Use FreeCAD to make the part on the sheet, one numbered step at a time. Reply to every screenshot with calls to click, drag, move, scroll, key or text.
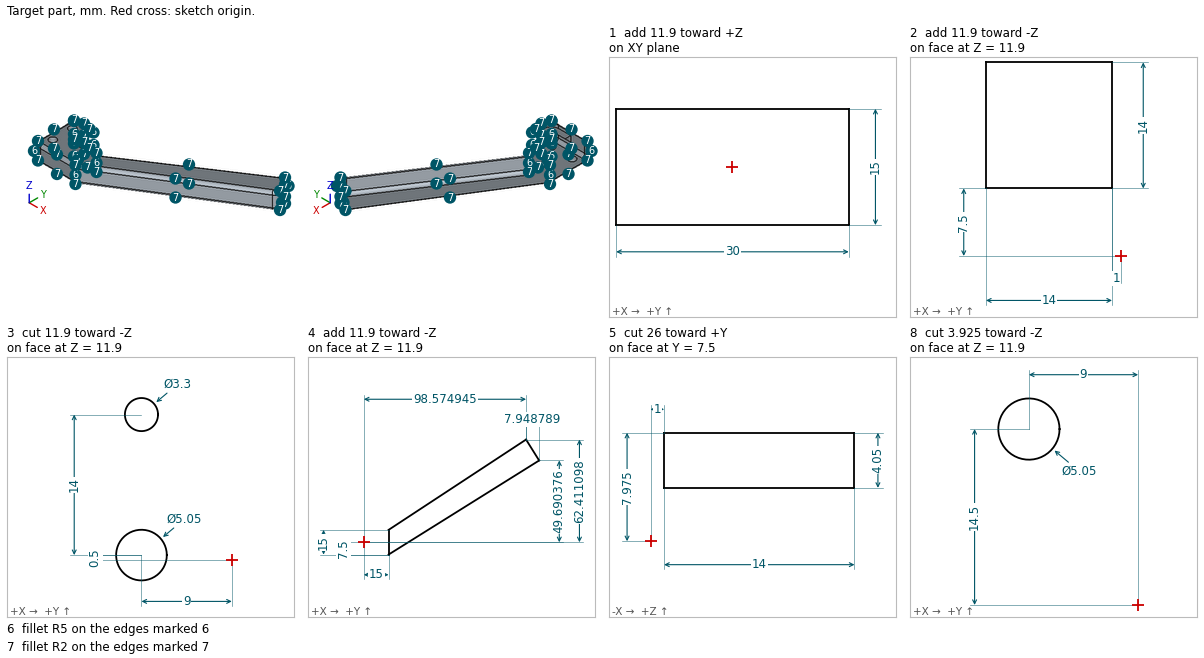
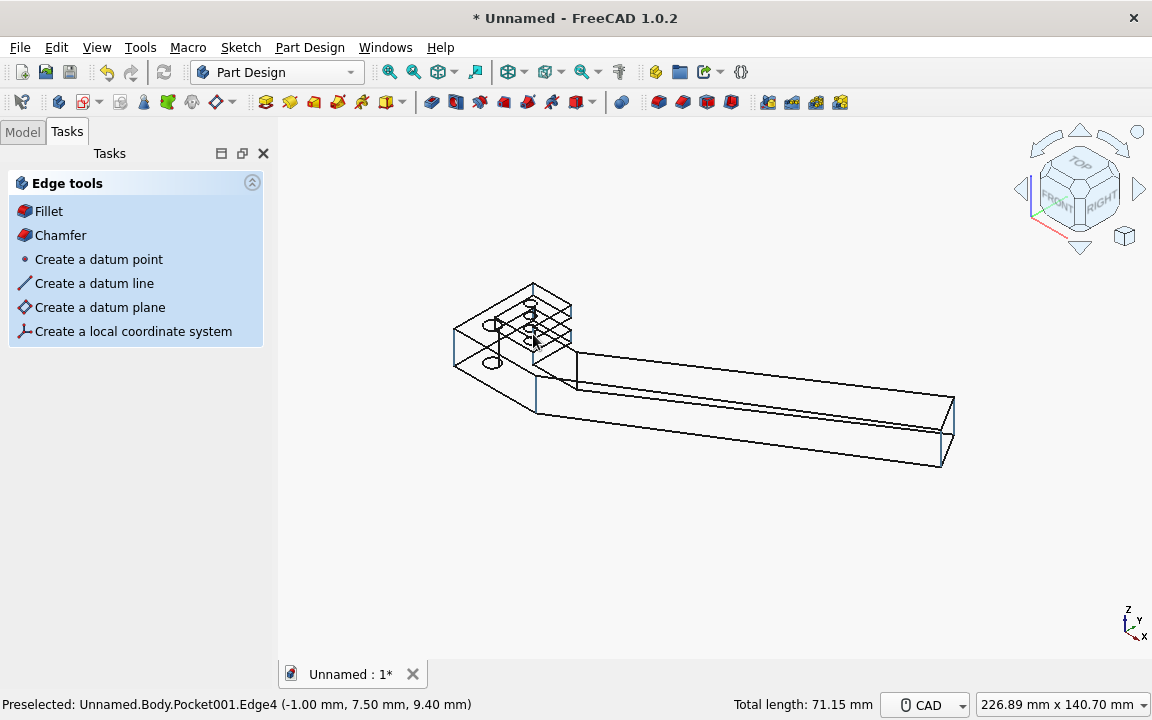
click(577, 370, ctrl)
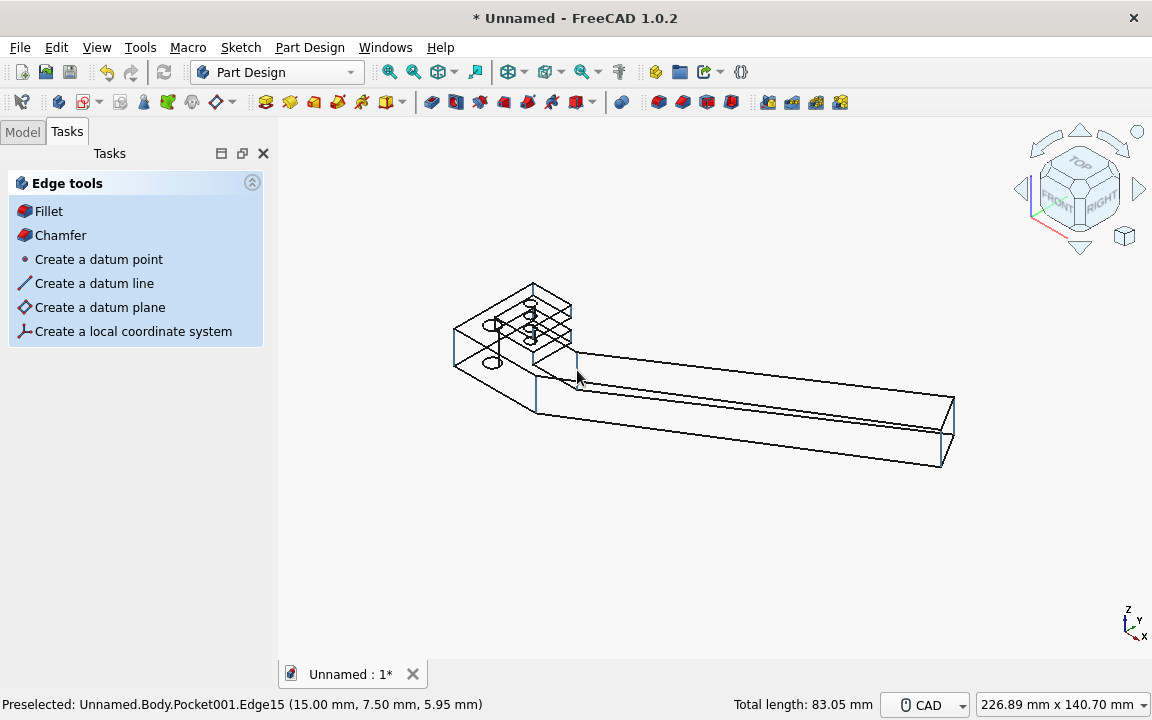
key(v)
key(1)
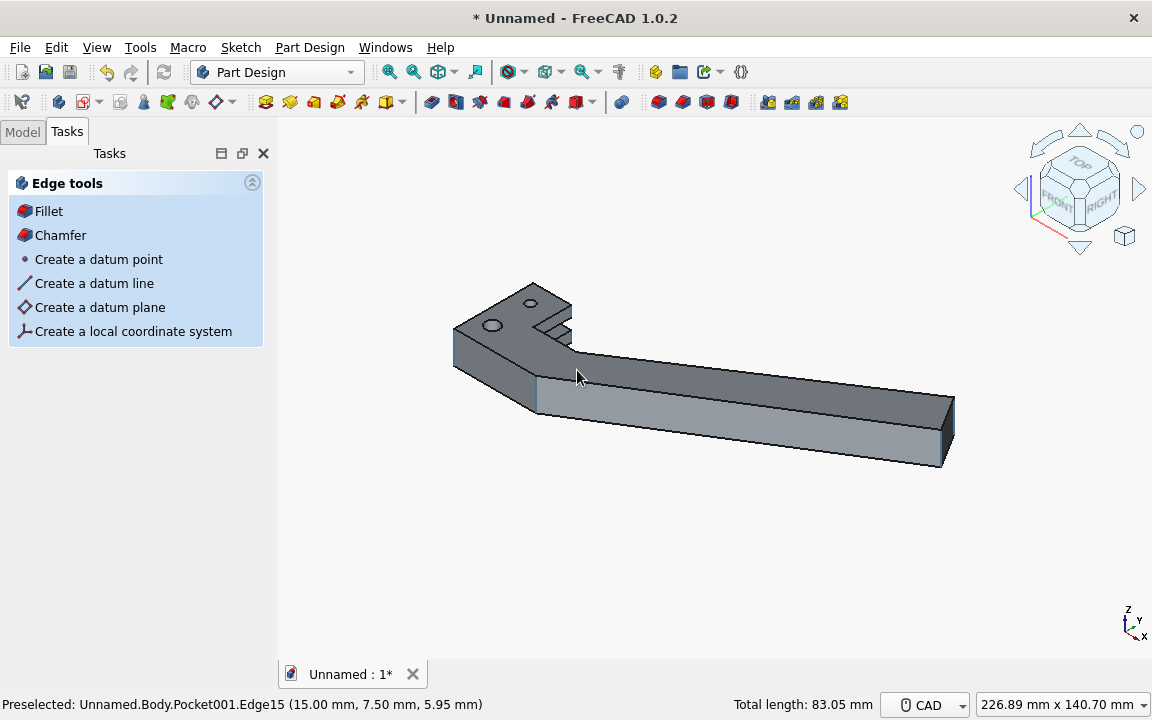
click(660, 102)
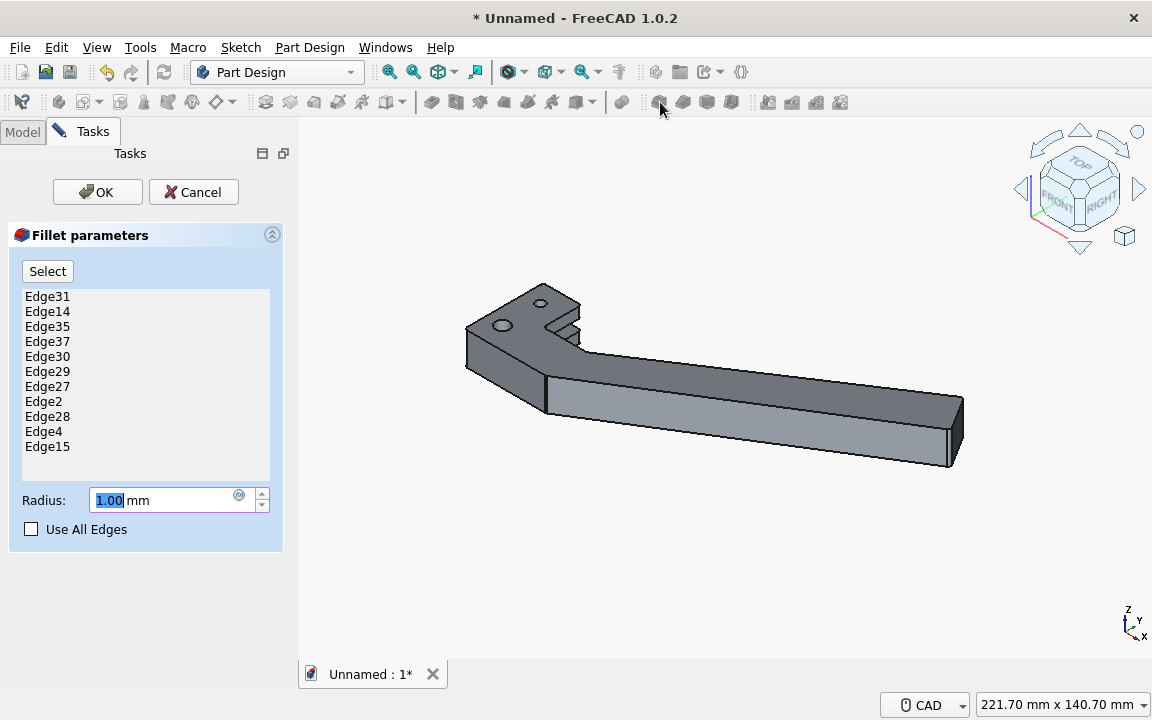
text(5)
key(Tab)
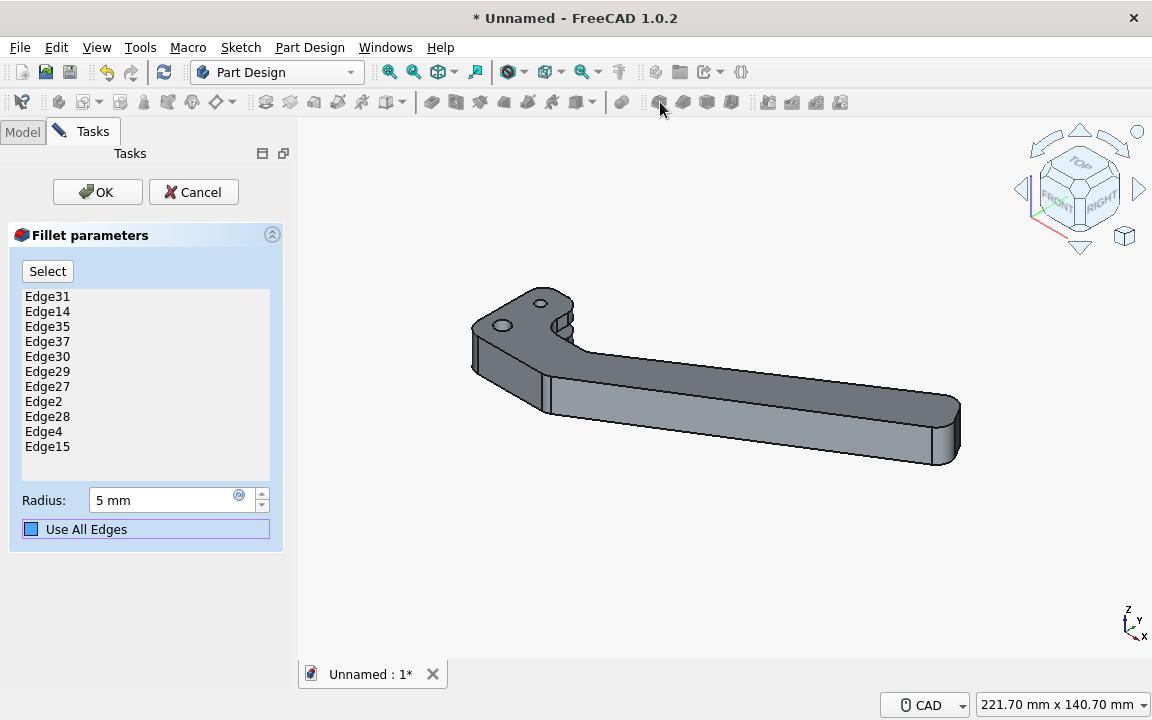
click(98, 192)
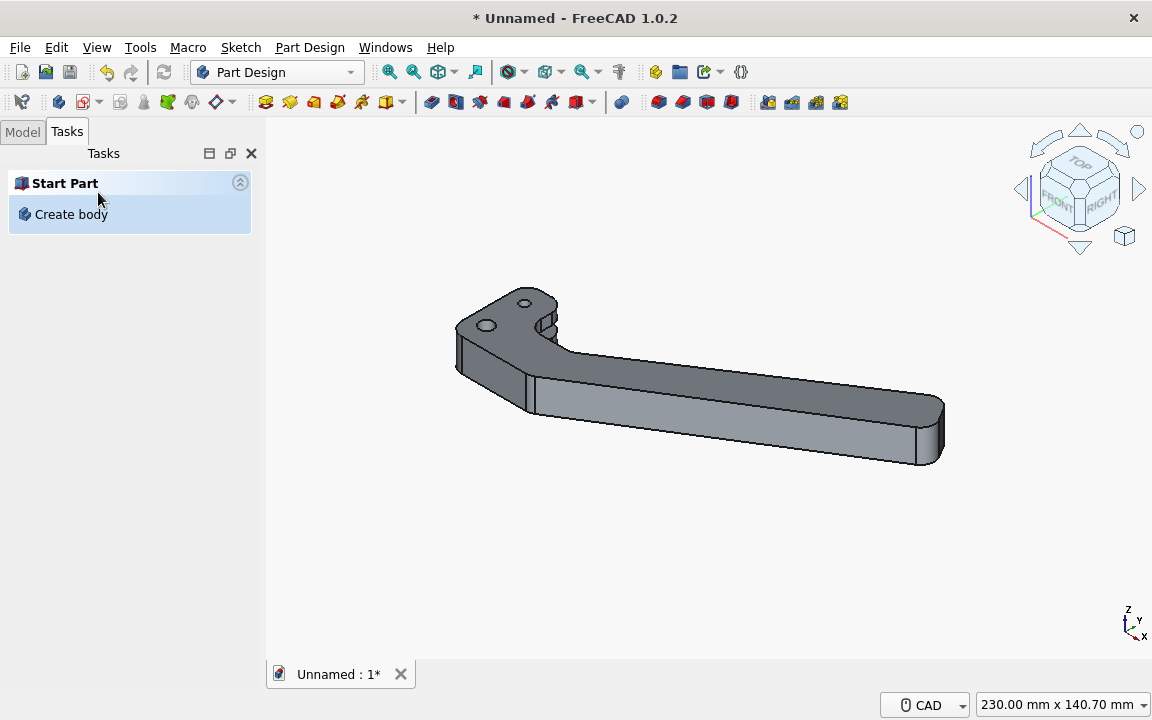
click(568, 349)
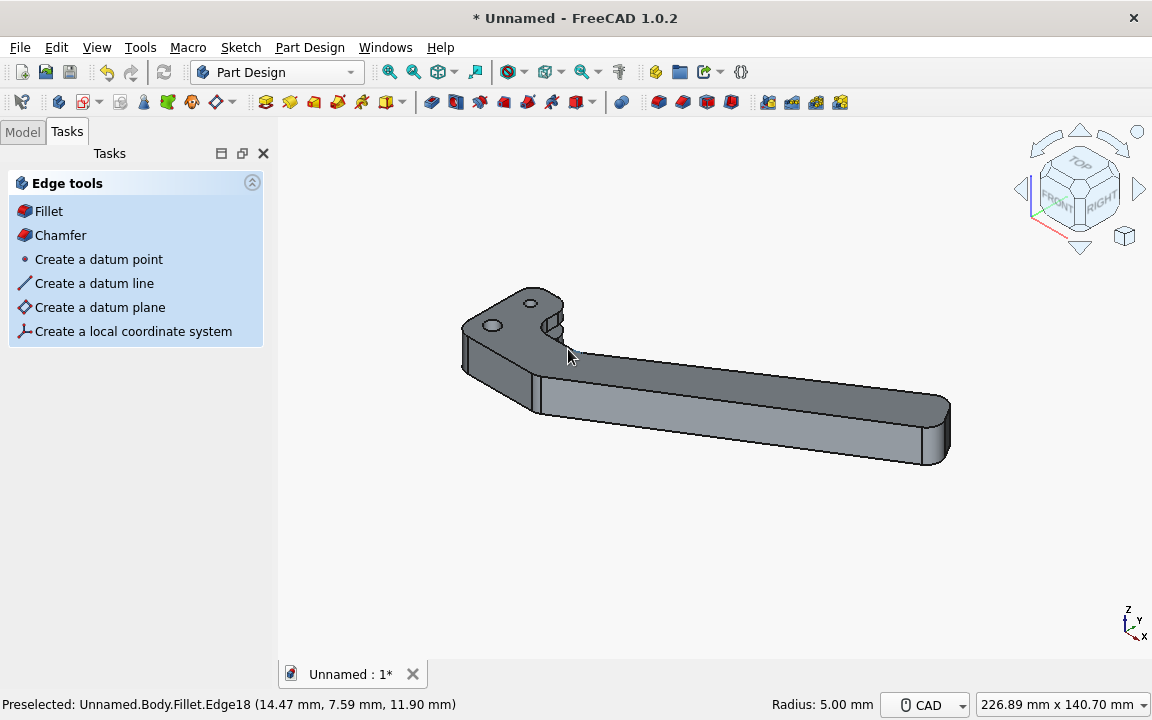
click(541, 326, ctrl)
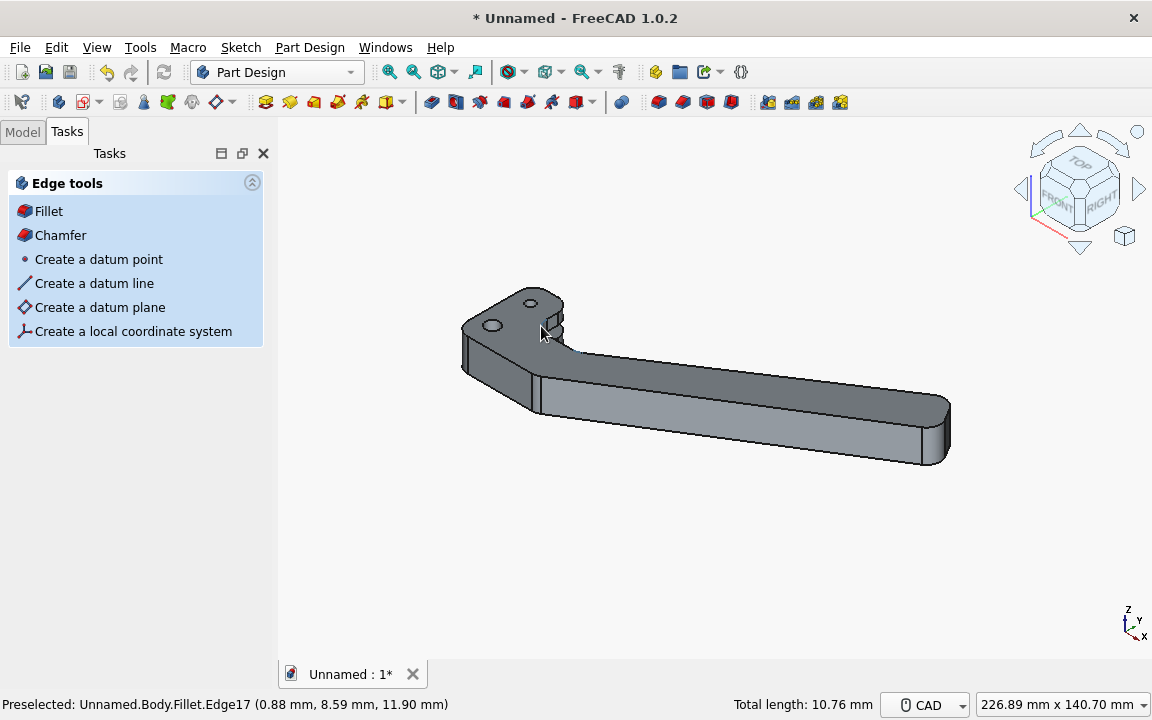
click(948, 412, ctrl)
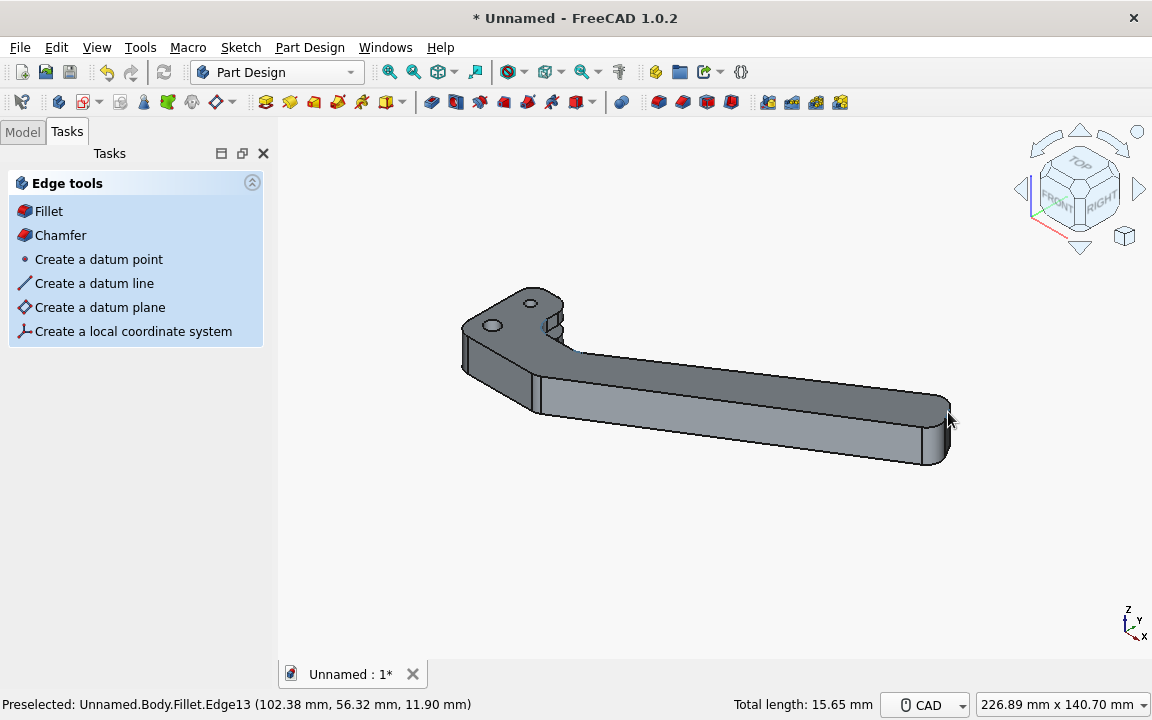
click(500, 354, ctrl)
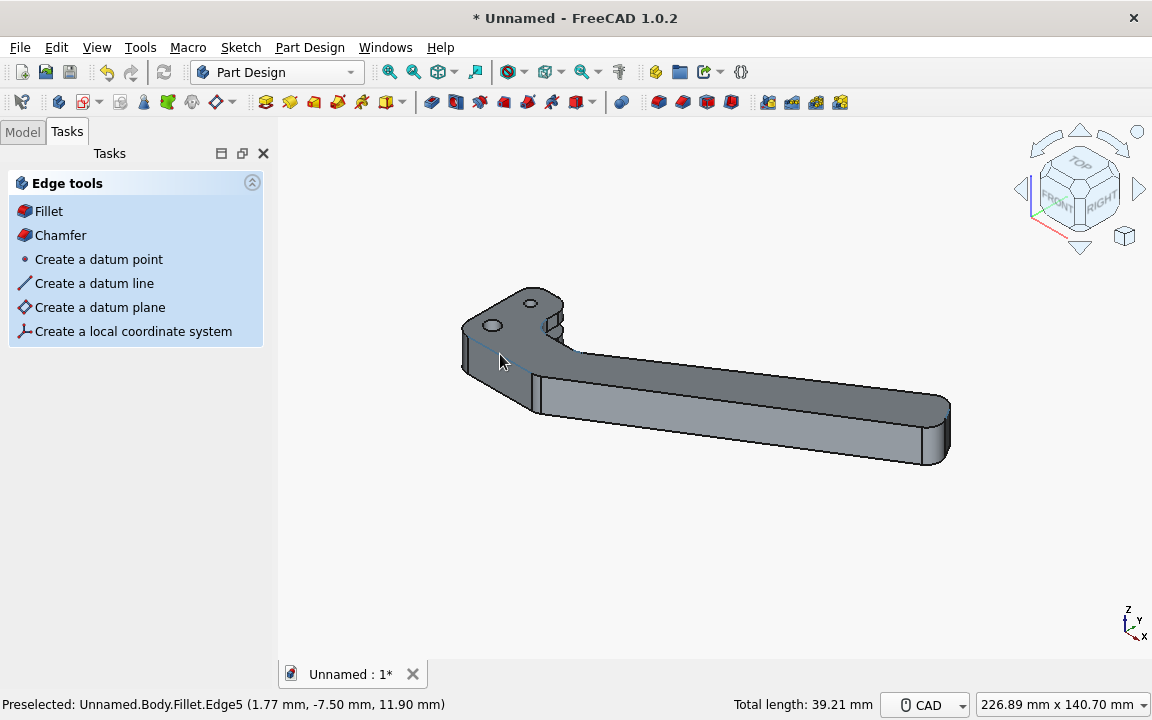
click(732, 401, ctrl)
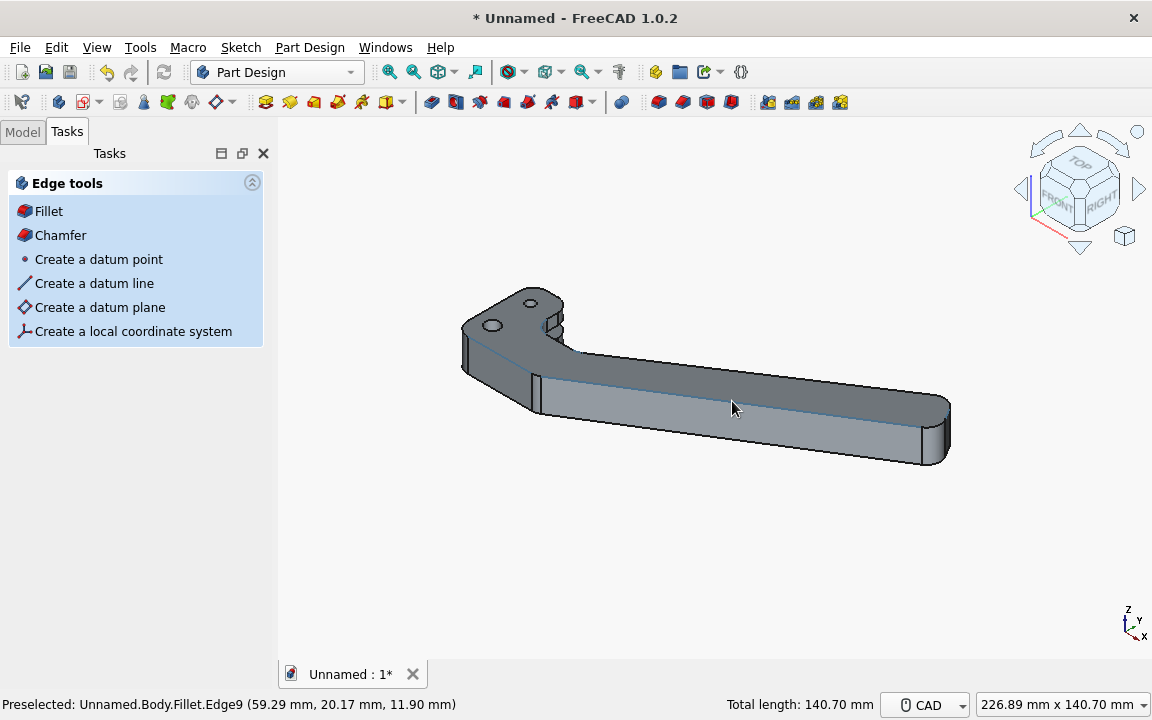
click(553, 314, ctrl)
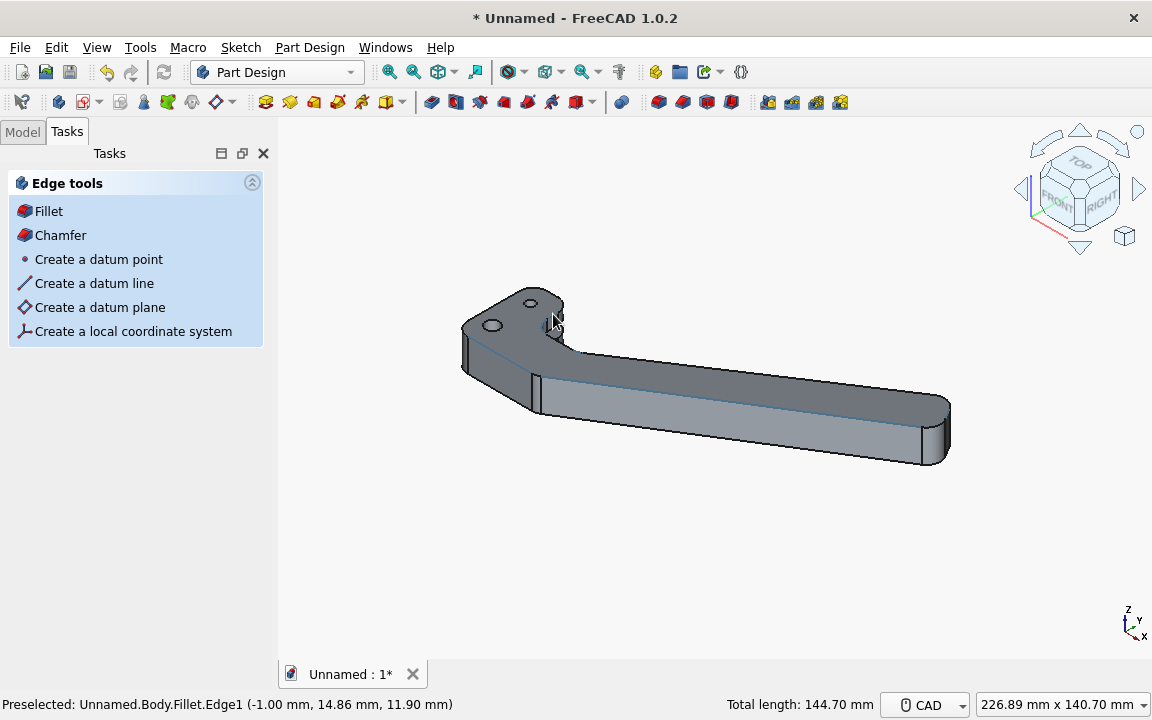
click(563, 304, ctrl)